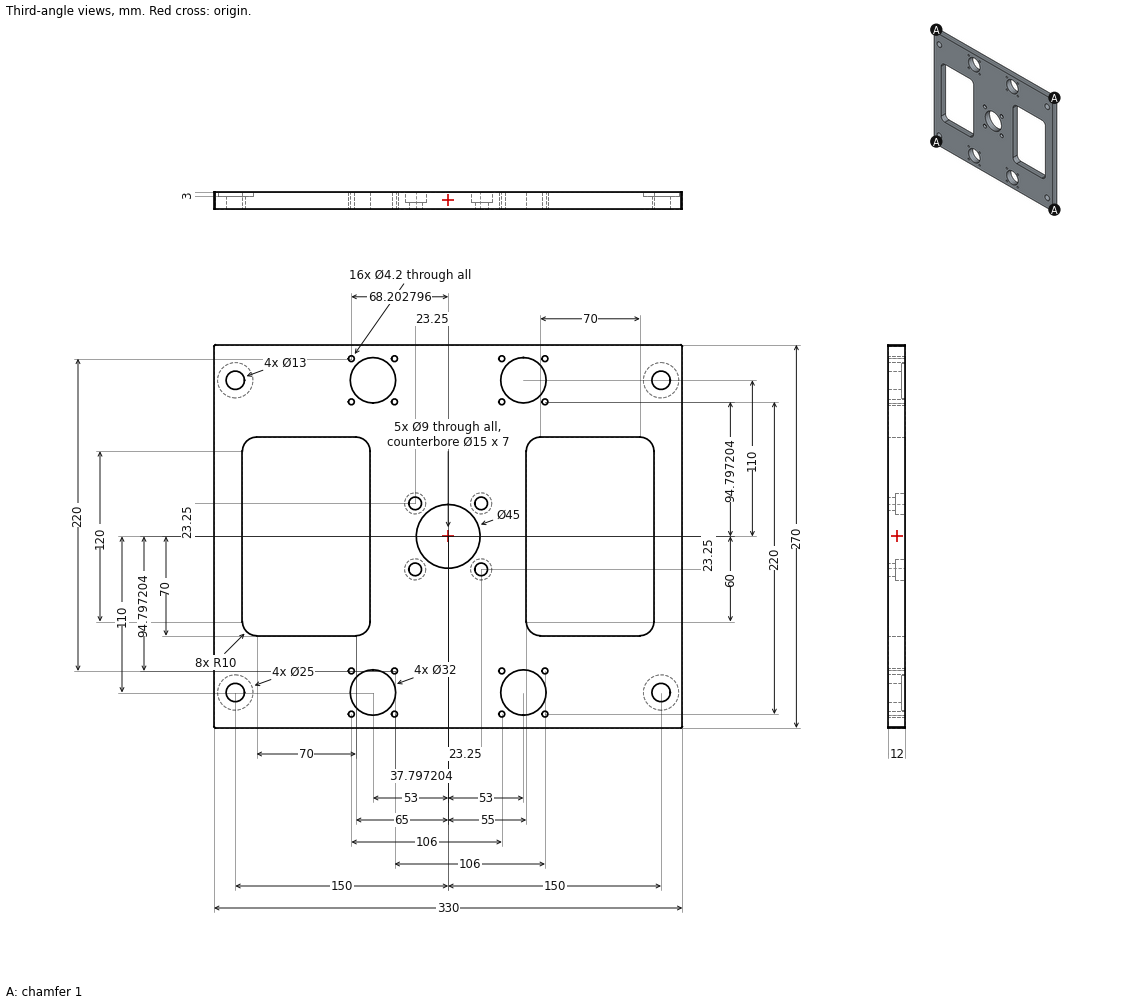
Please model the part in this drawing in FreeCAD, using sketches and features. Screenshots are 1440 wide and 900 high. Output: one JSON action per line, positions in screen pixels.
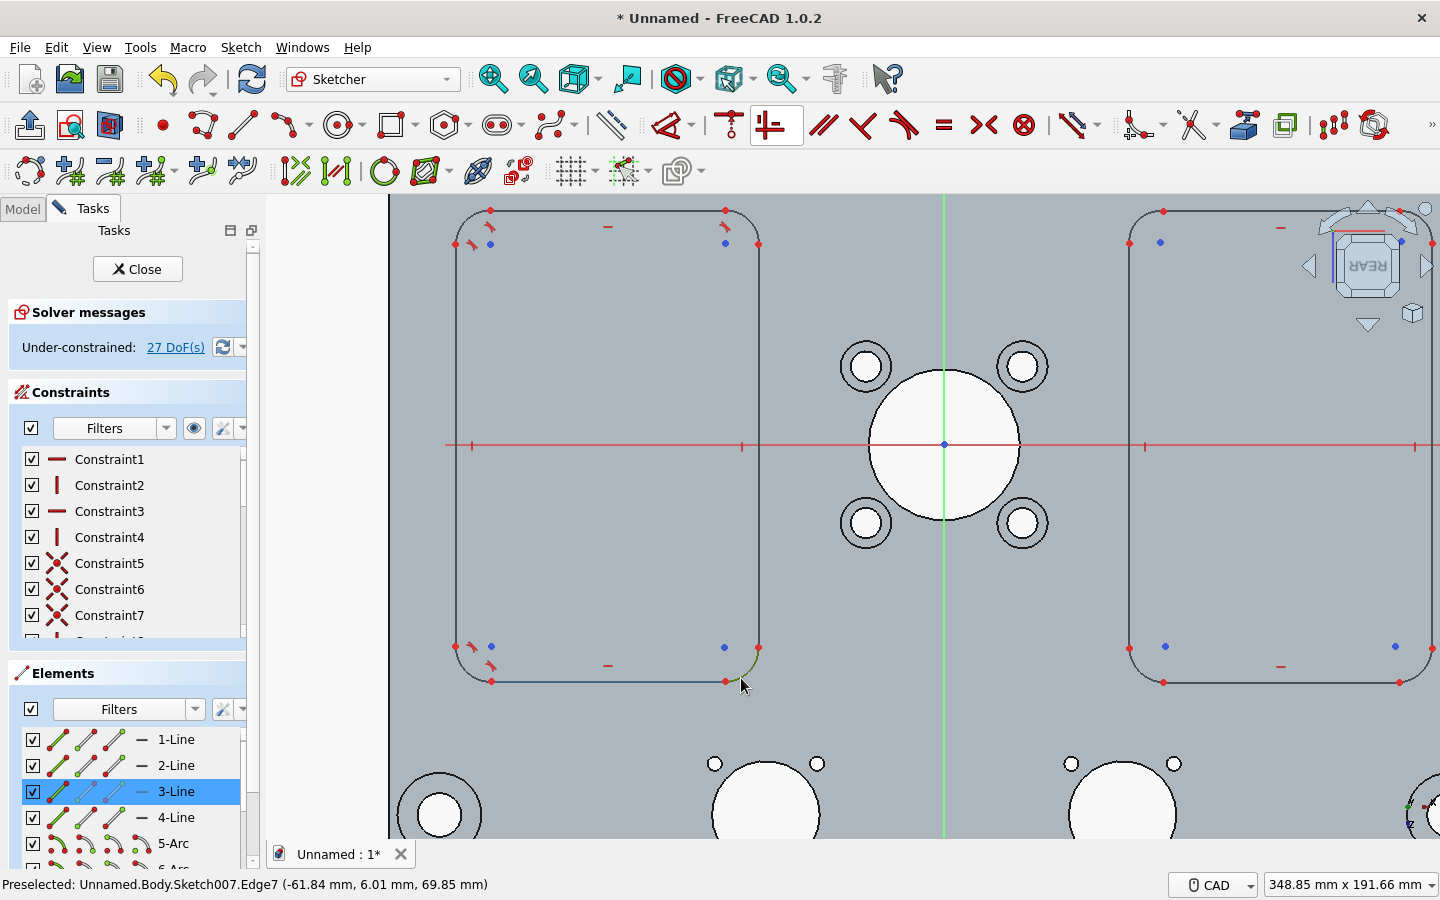
{"action": "left_click", "coordinate": [904, 126]}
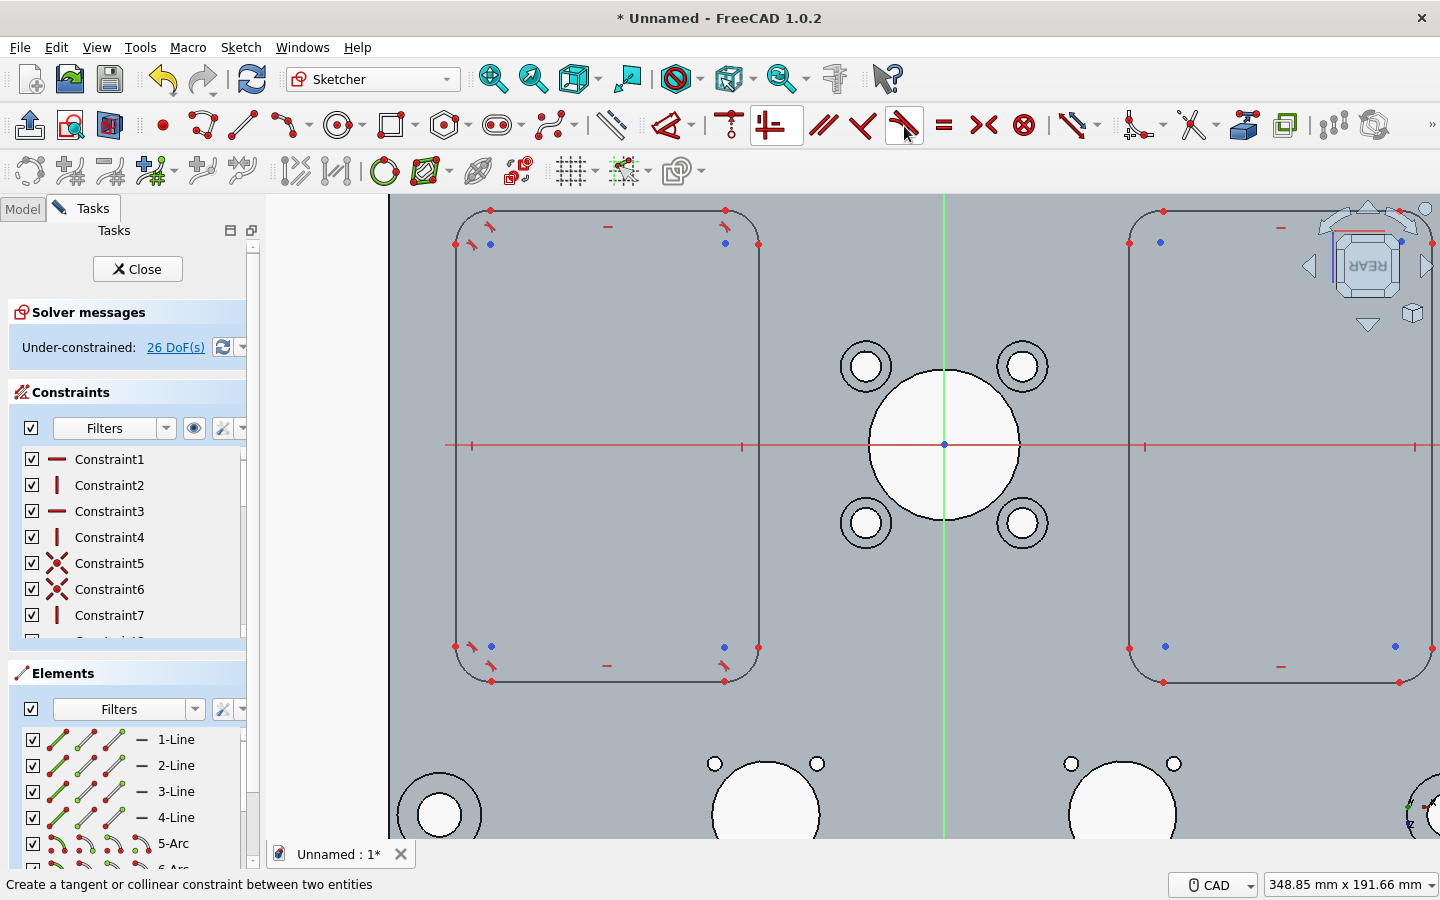
{"action": "left_click", "coordinate": [759, 527]}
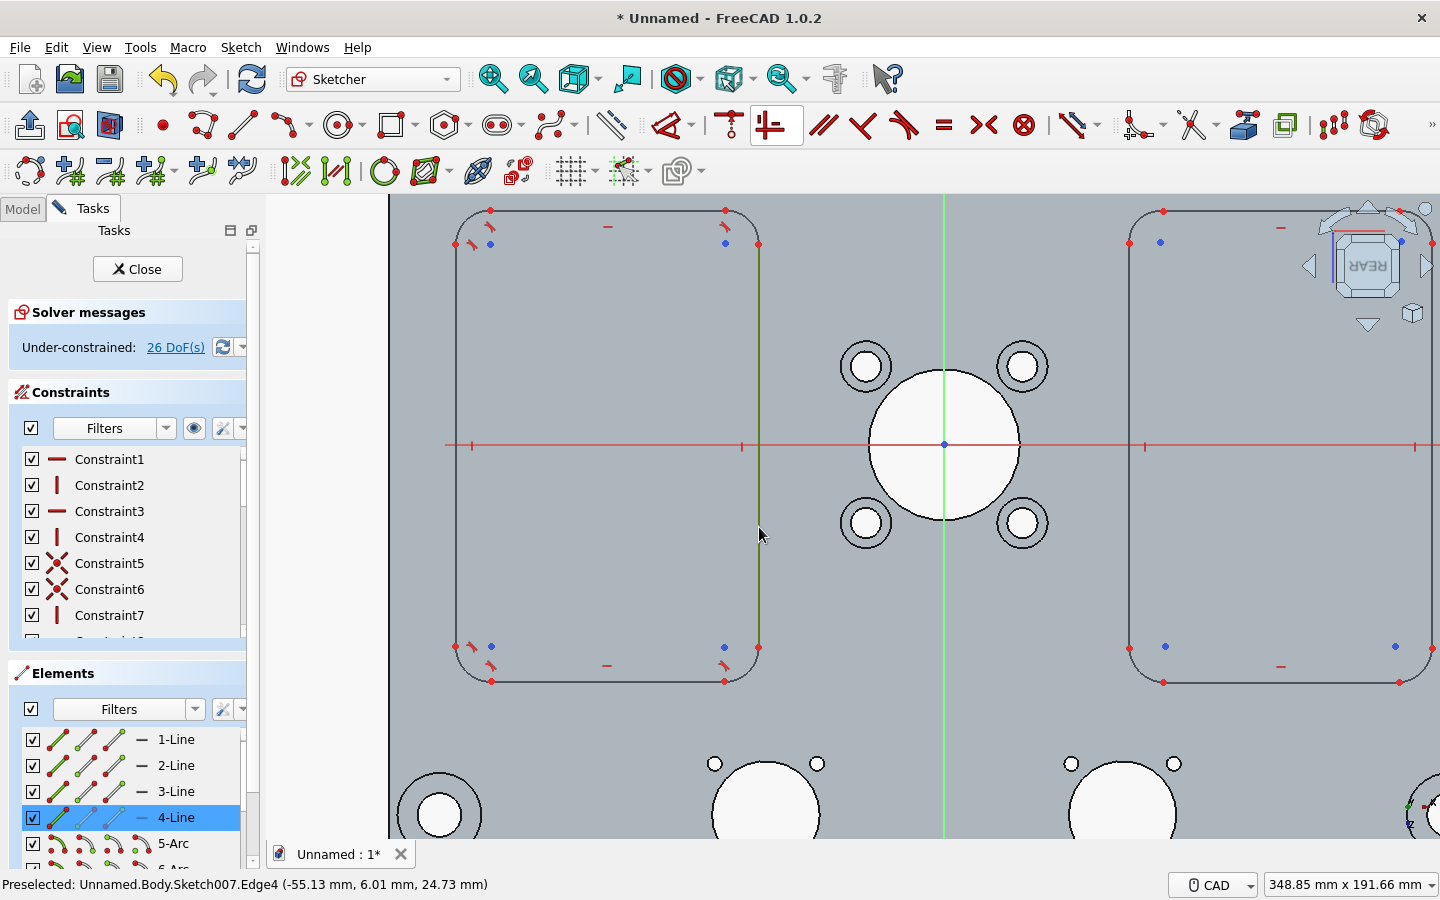
{"action": "left_click", "coordinate": [740, 678]}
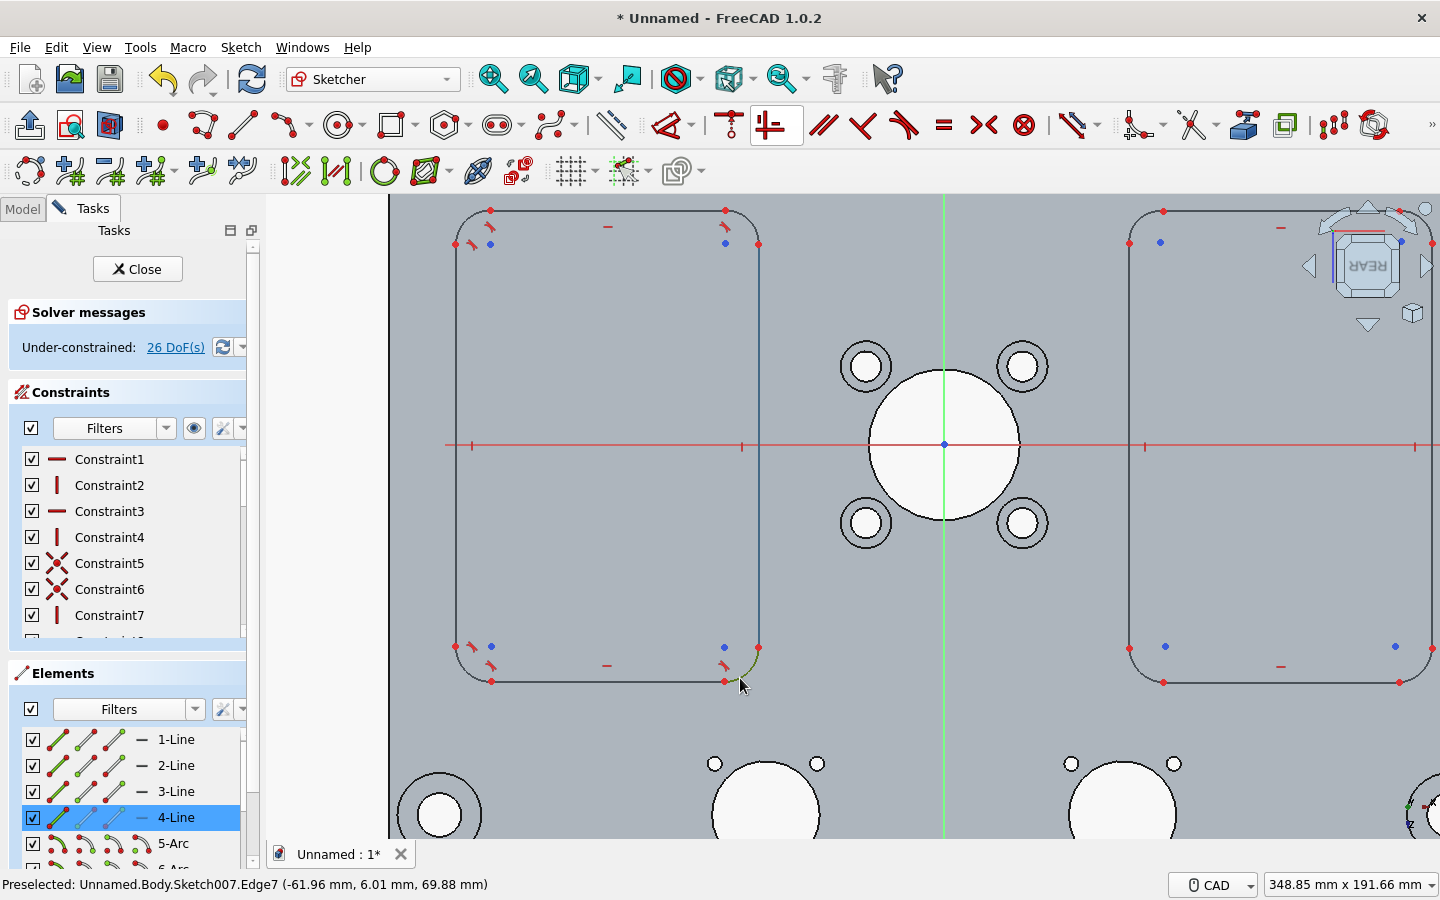
{"action": "key", "text": "t"}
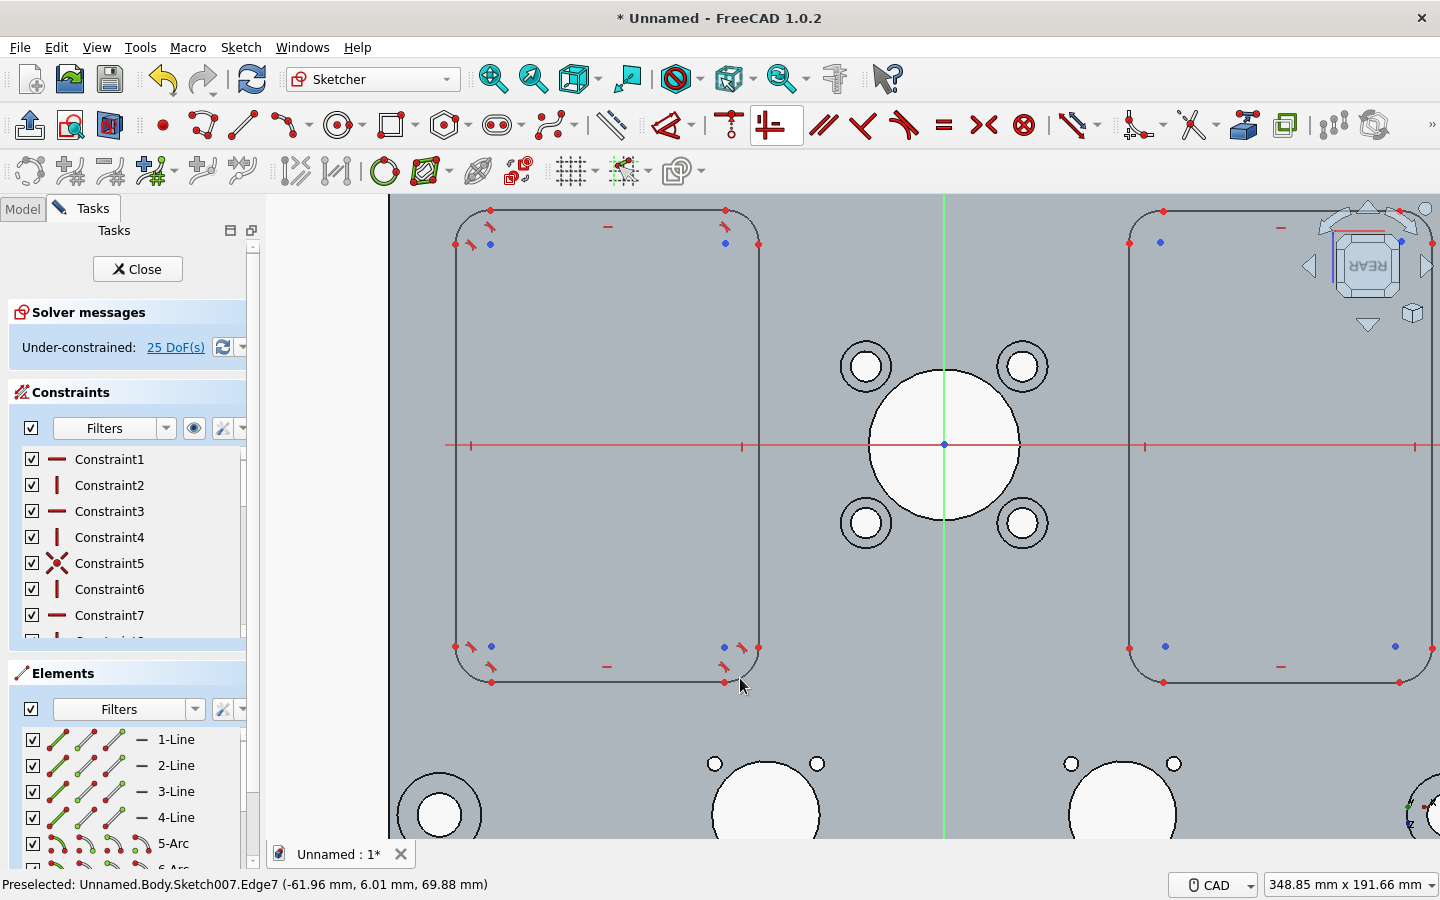
{"action": "left_click", "coordinate": [759, 527]}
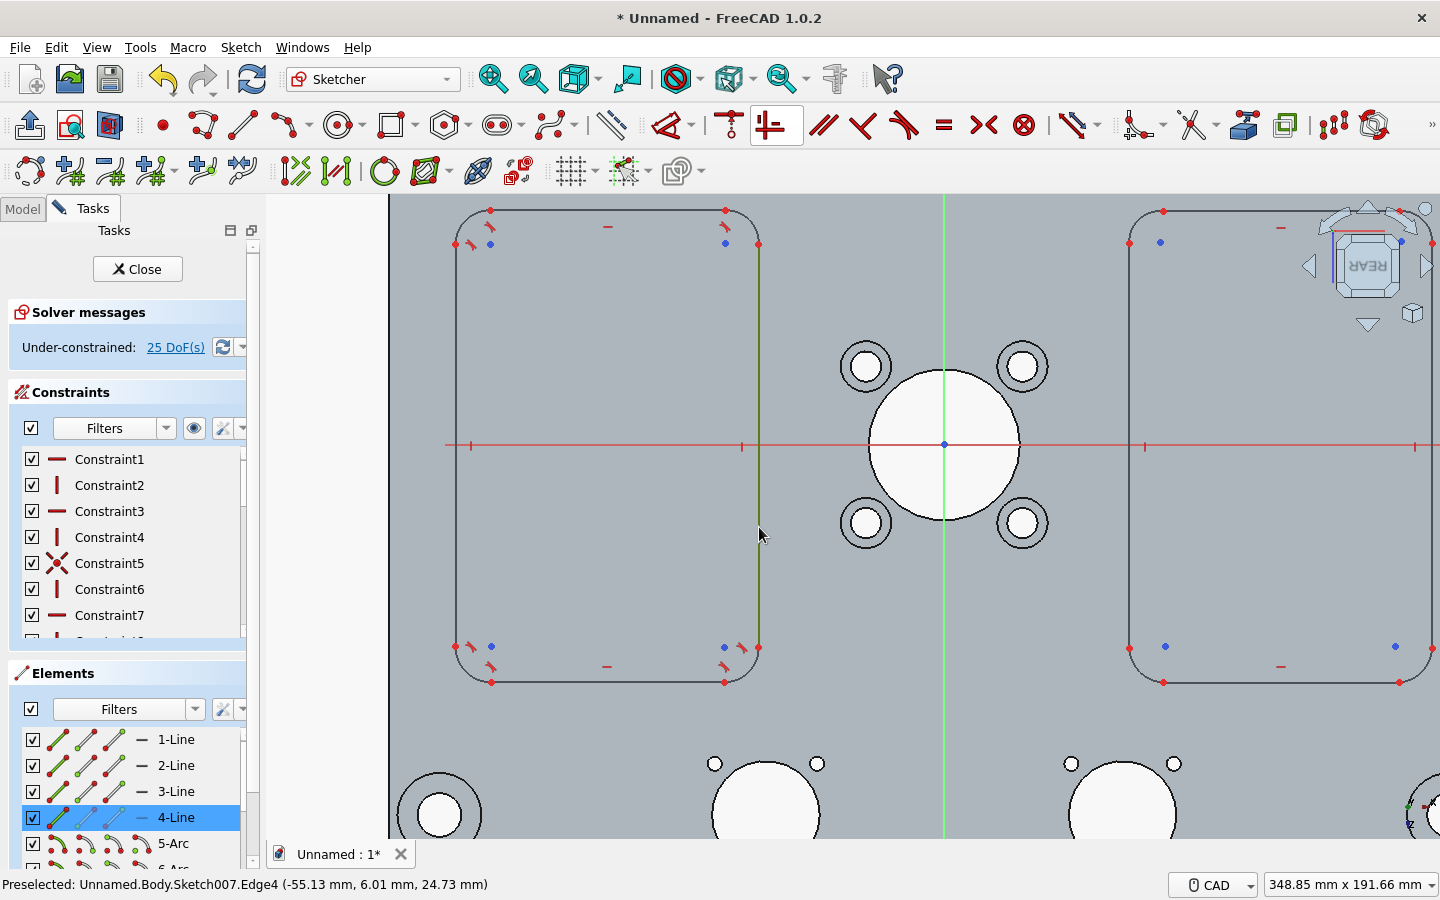
{"action": "left_click", "coordinate": [756, 229]}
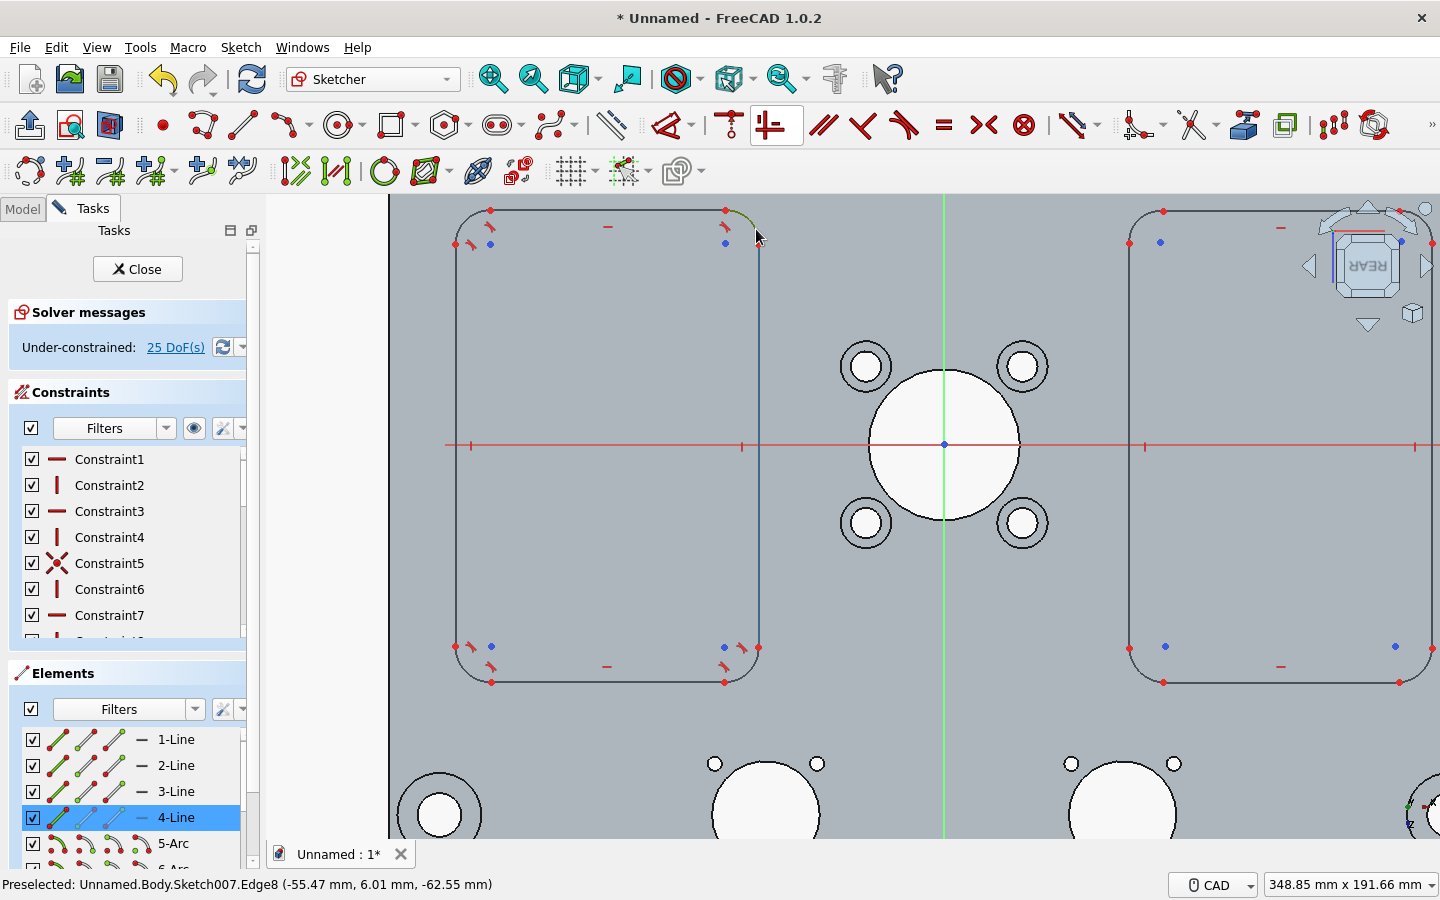
{"action": "left_click", "coordinate": [904, 126]}